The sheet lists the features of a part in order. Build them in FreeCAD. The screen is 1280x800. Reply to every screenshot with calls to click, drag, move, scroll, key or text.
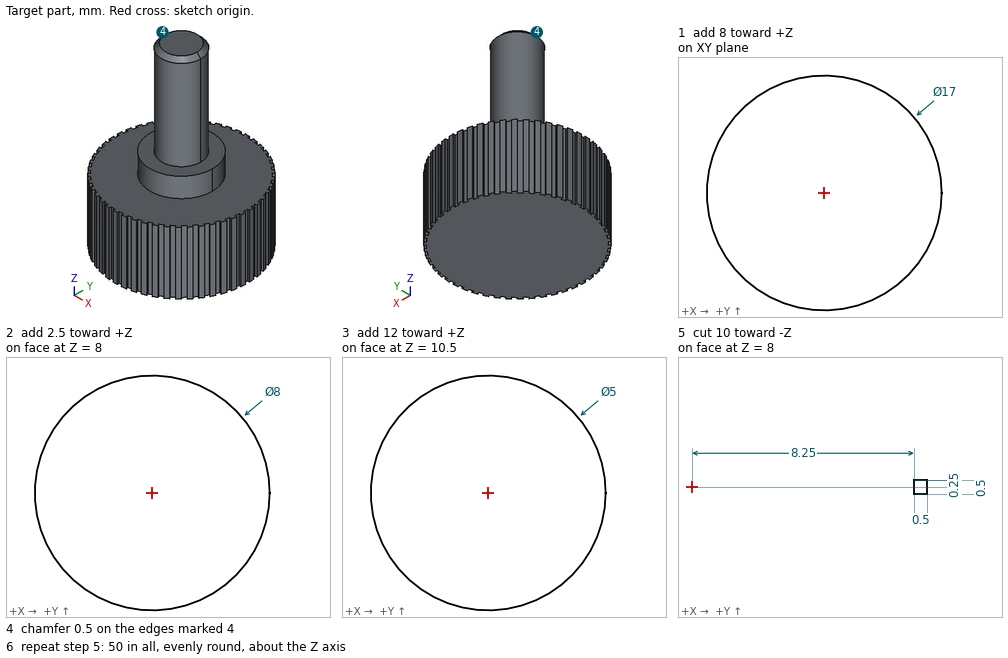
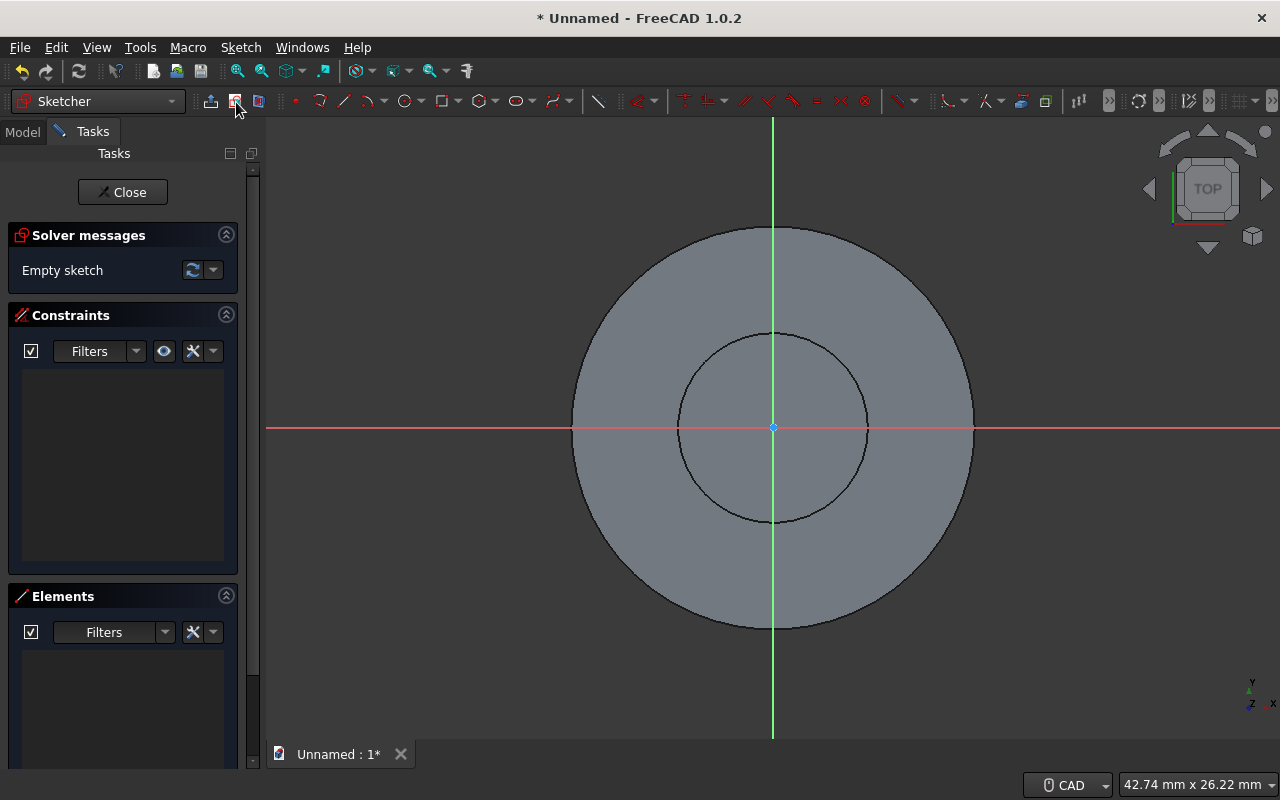
scroll(803, 428, up, 6)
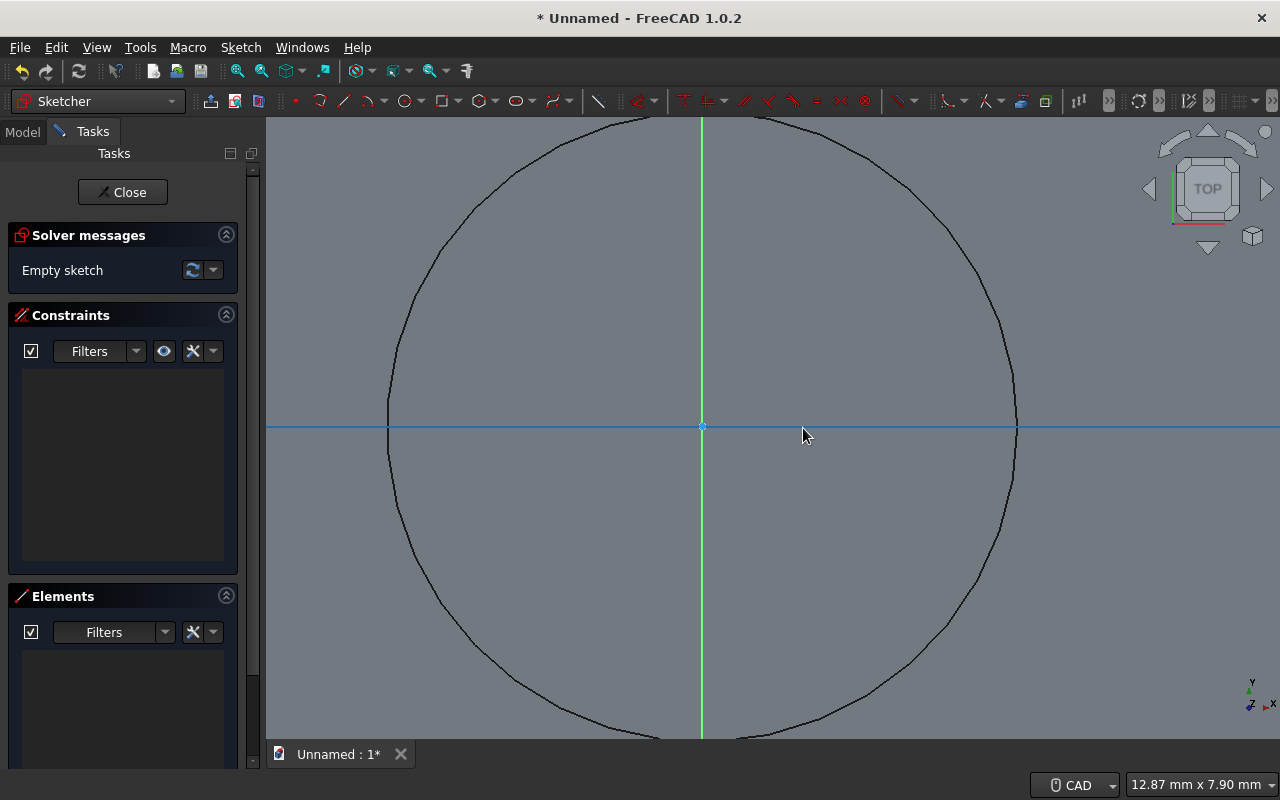
key(g)
key(c)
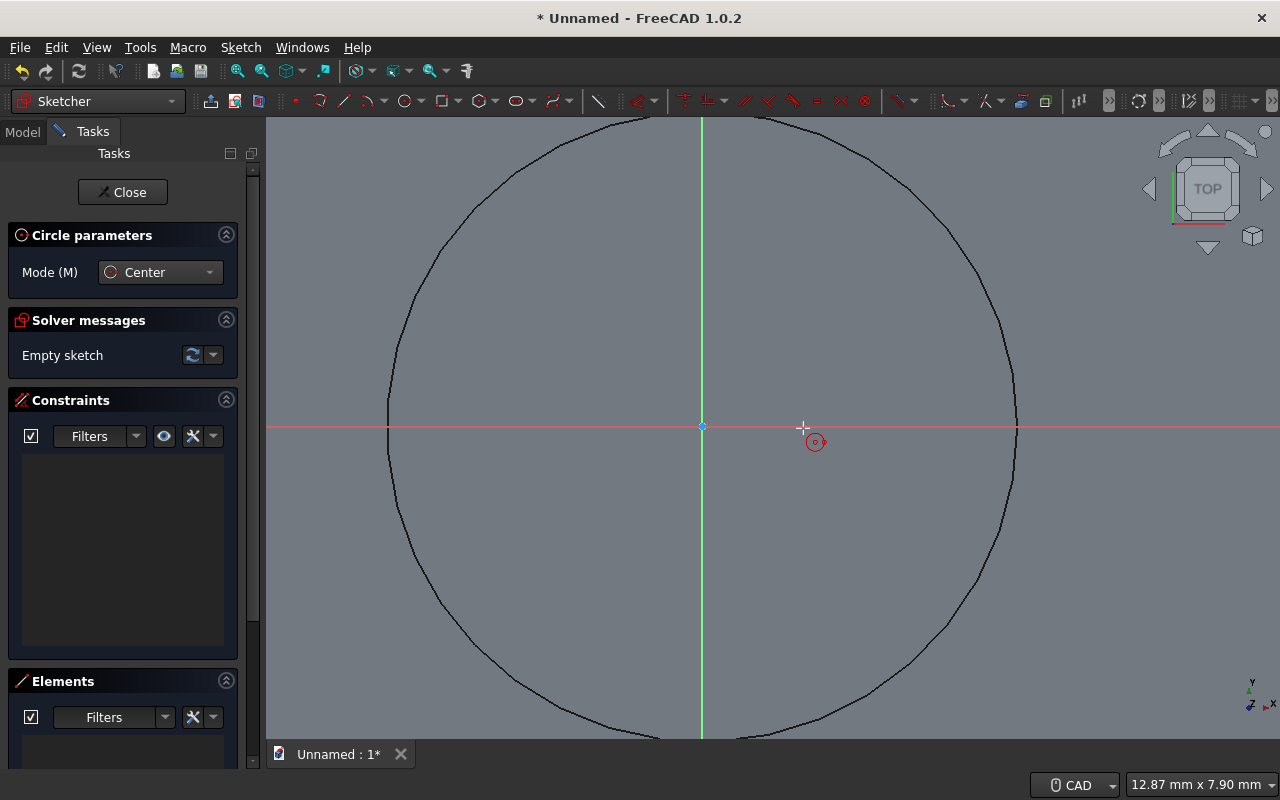
click(702, 427)
click(841, 288)
key(Escape)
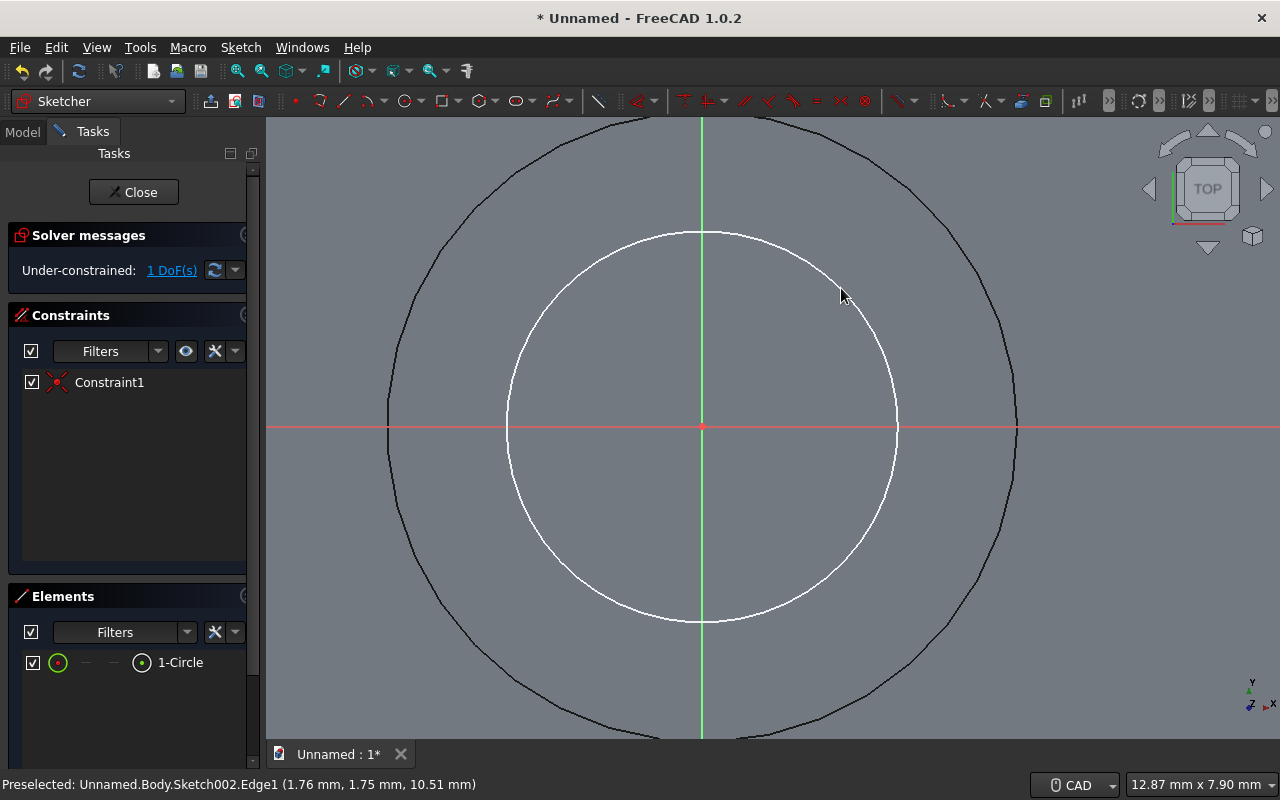
key(d)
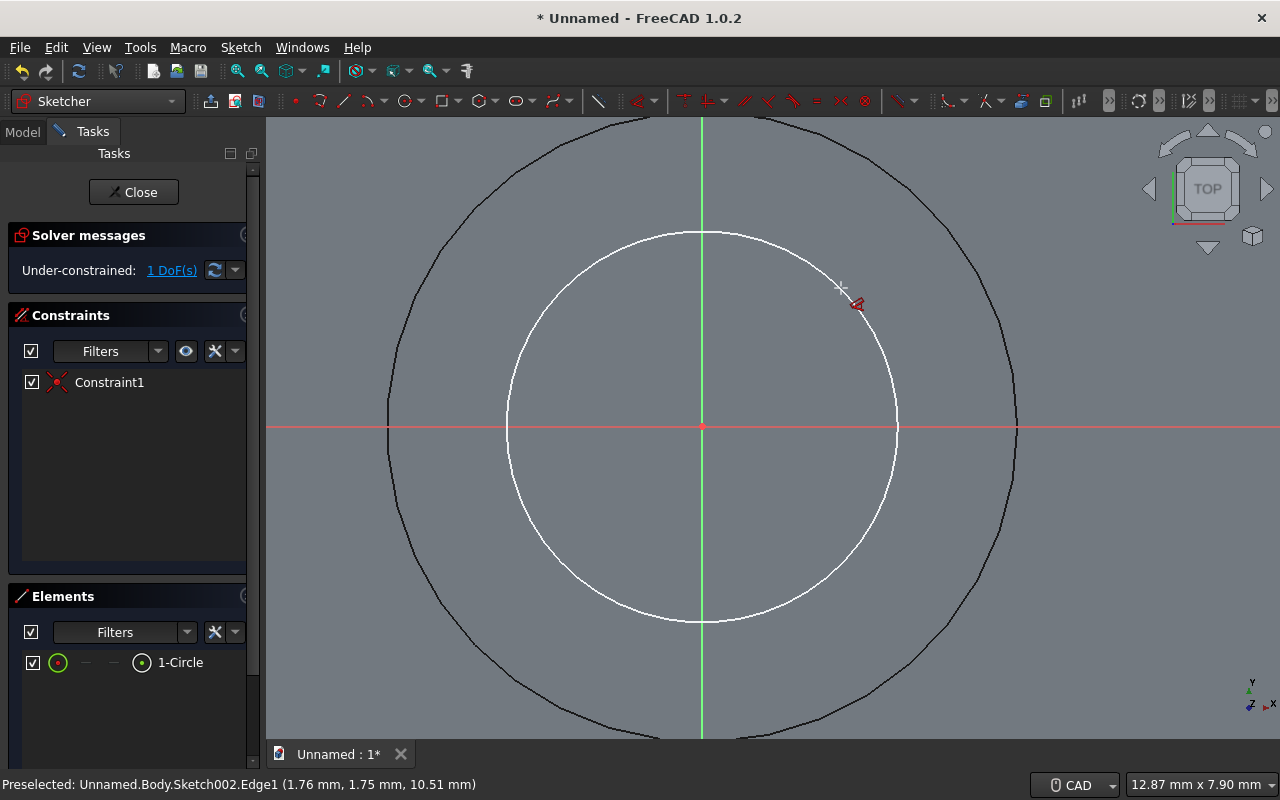
click(840, 288)
click(863, 265)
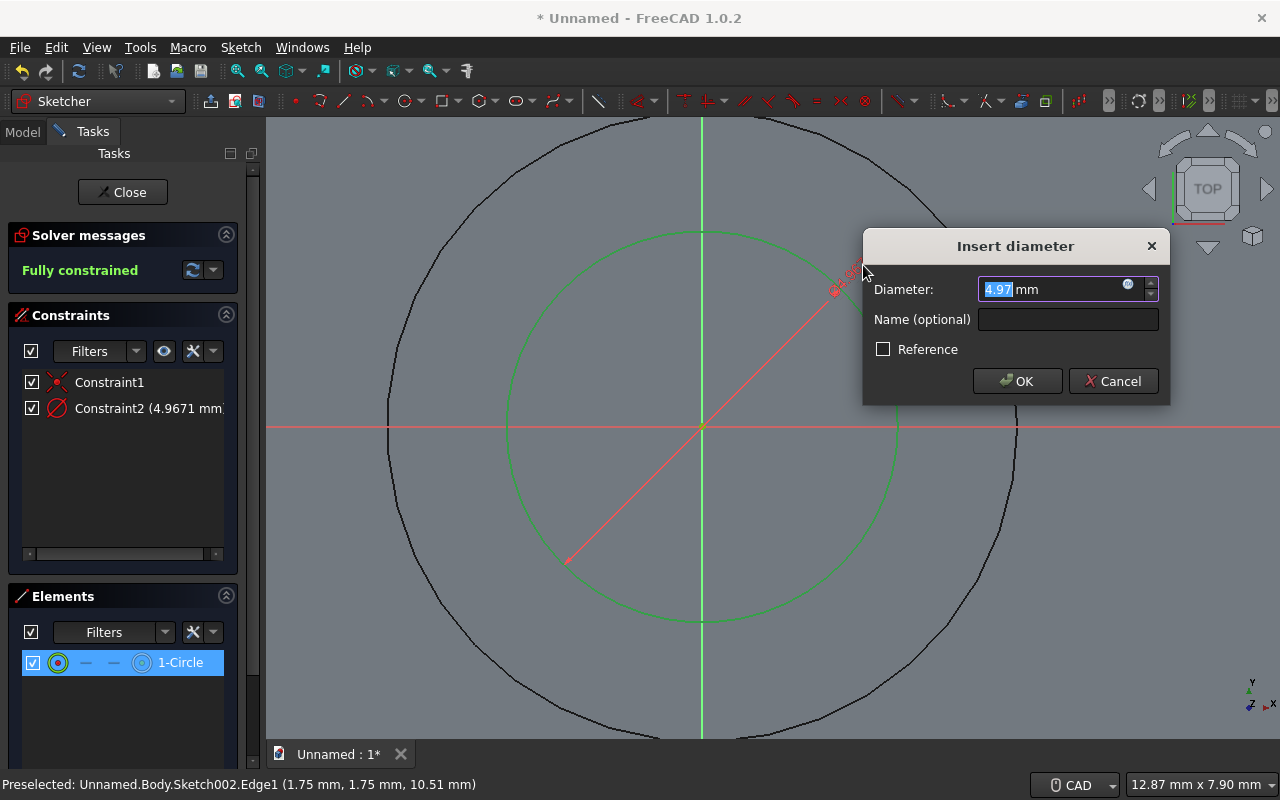
text(5)
key(Return)
key(Escape)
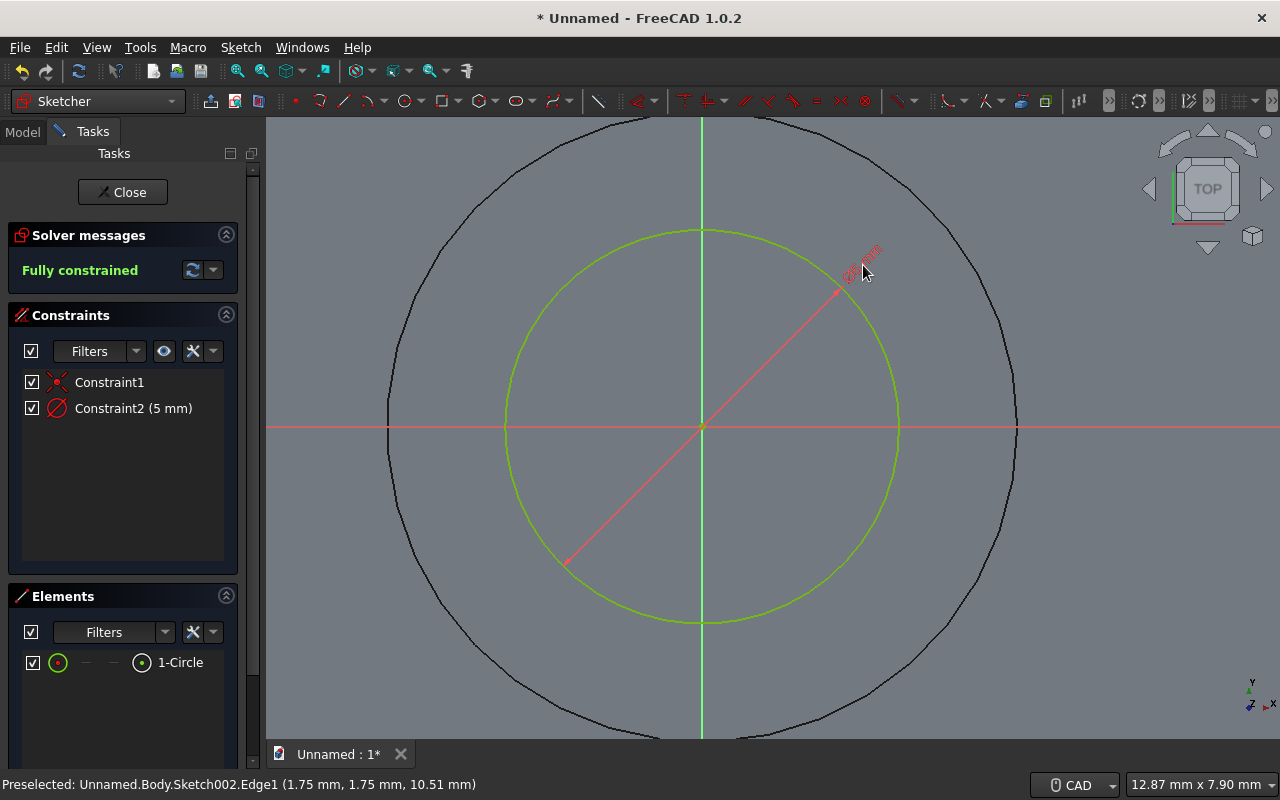
click(123, 192)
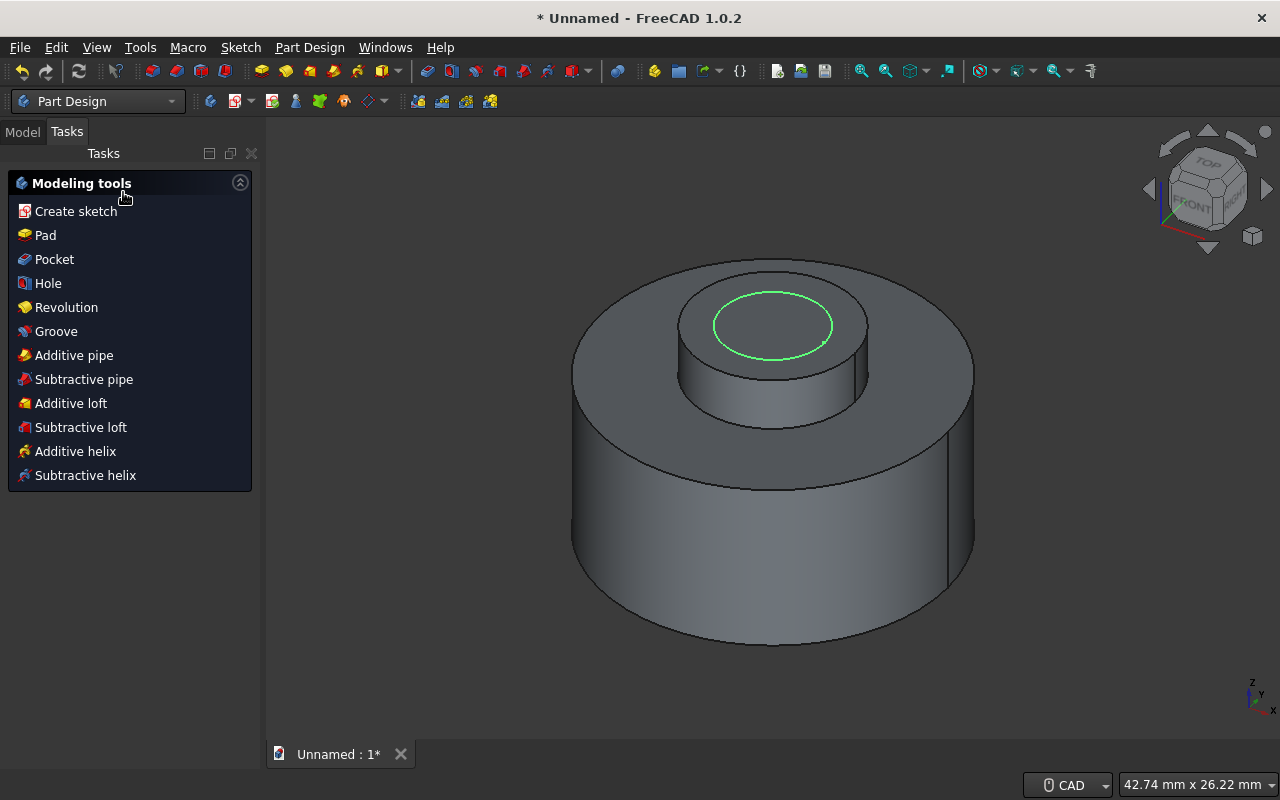
click(262, 72)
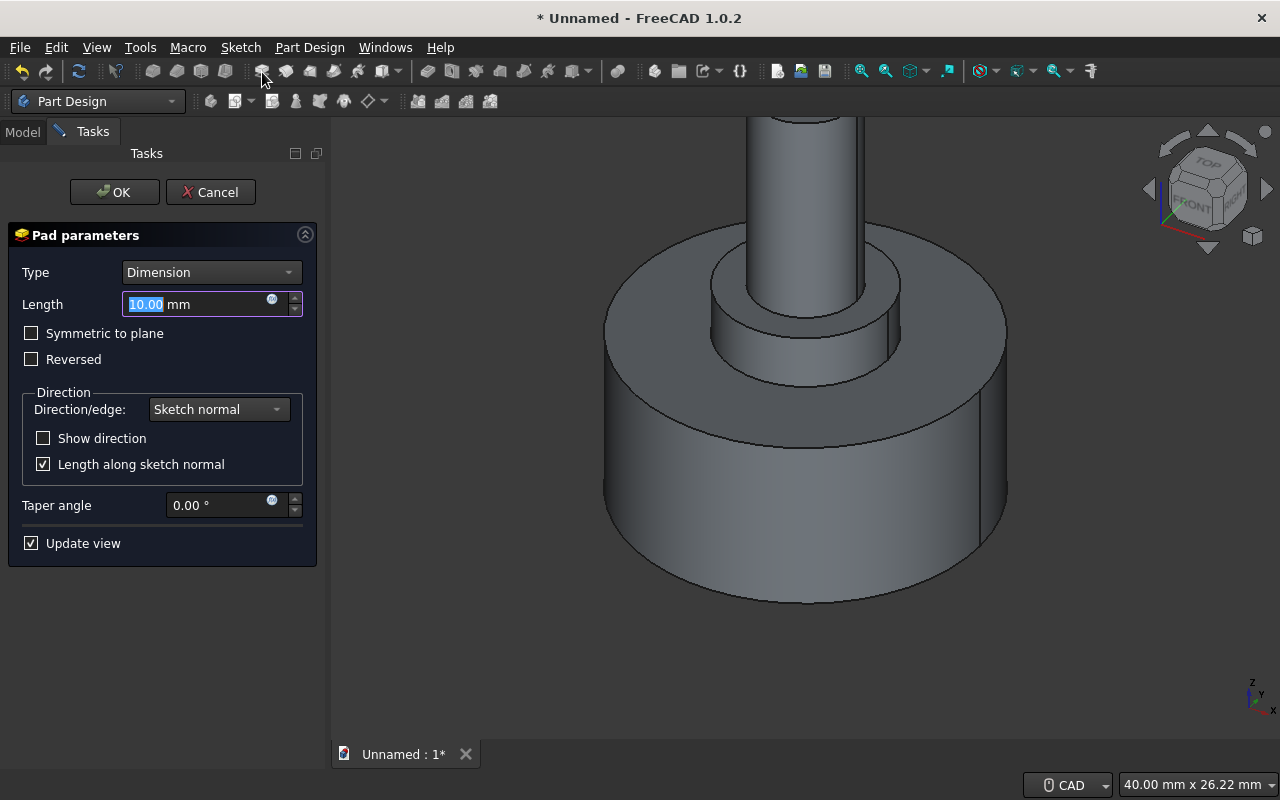
text(12)
key(Tab)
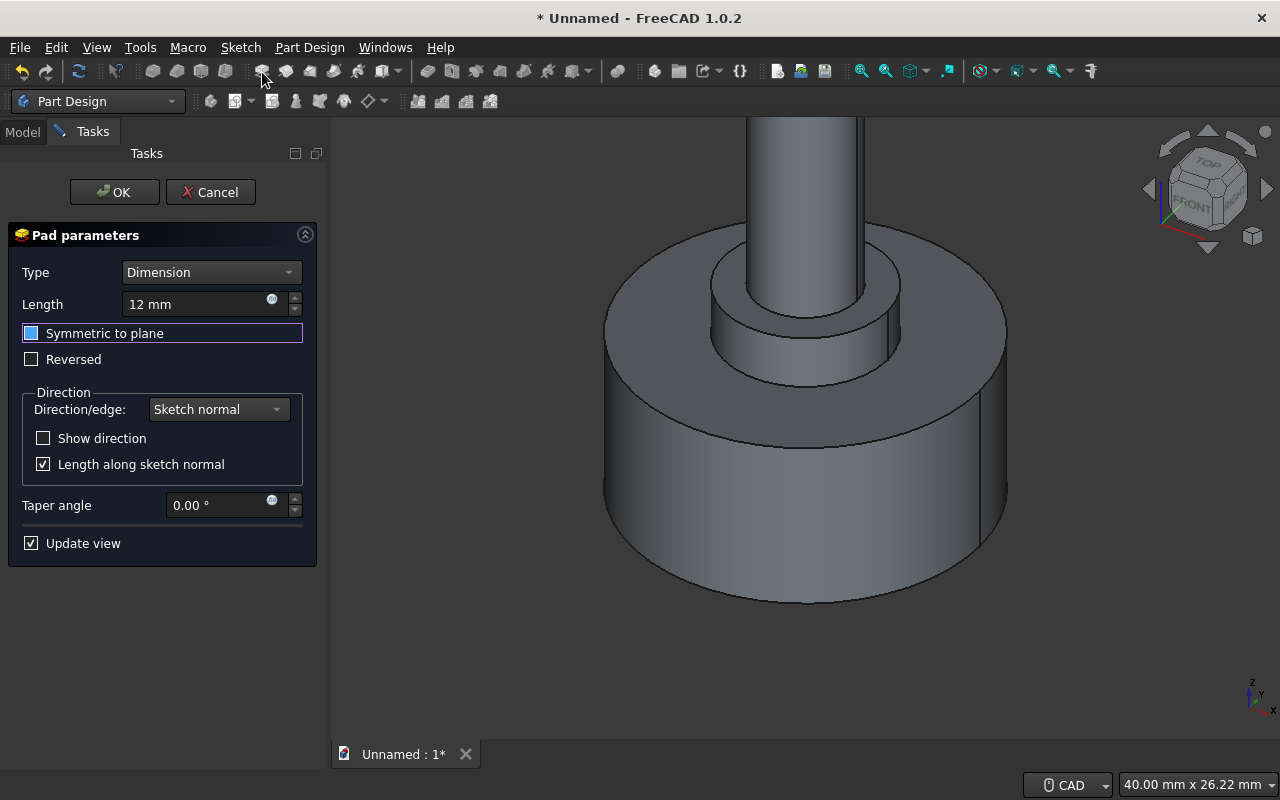
click(115, 192)